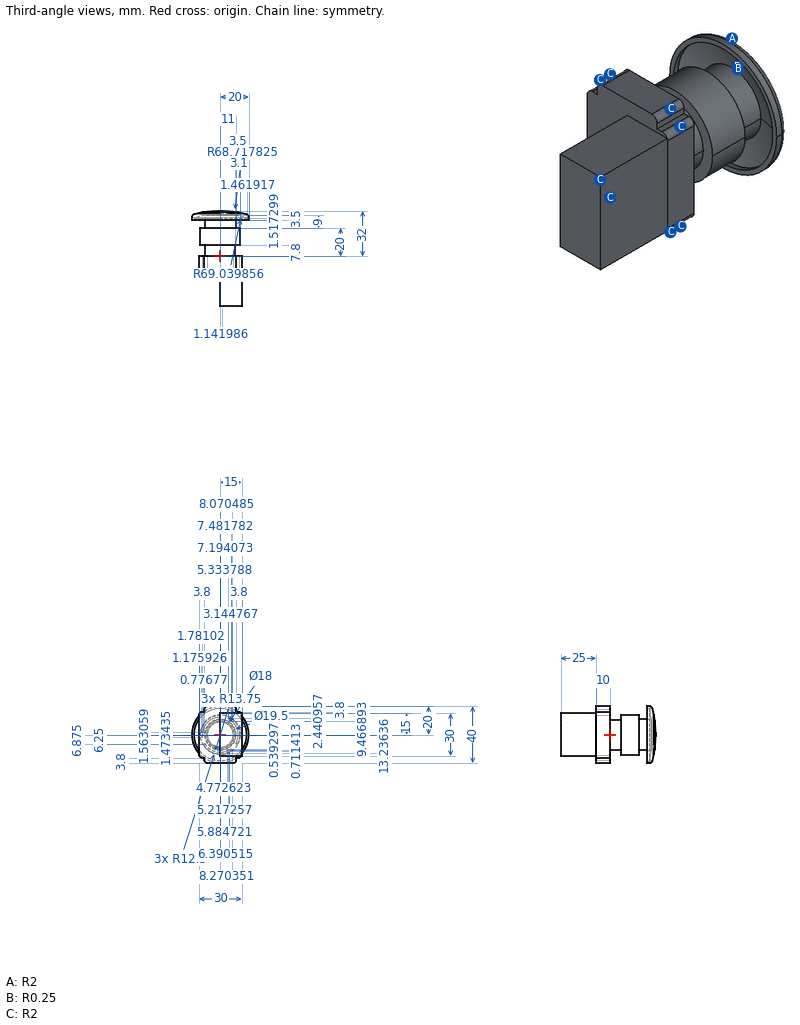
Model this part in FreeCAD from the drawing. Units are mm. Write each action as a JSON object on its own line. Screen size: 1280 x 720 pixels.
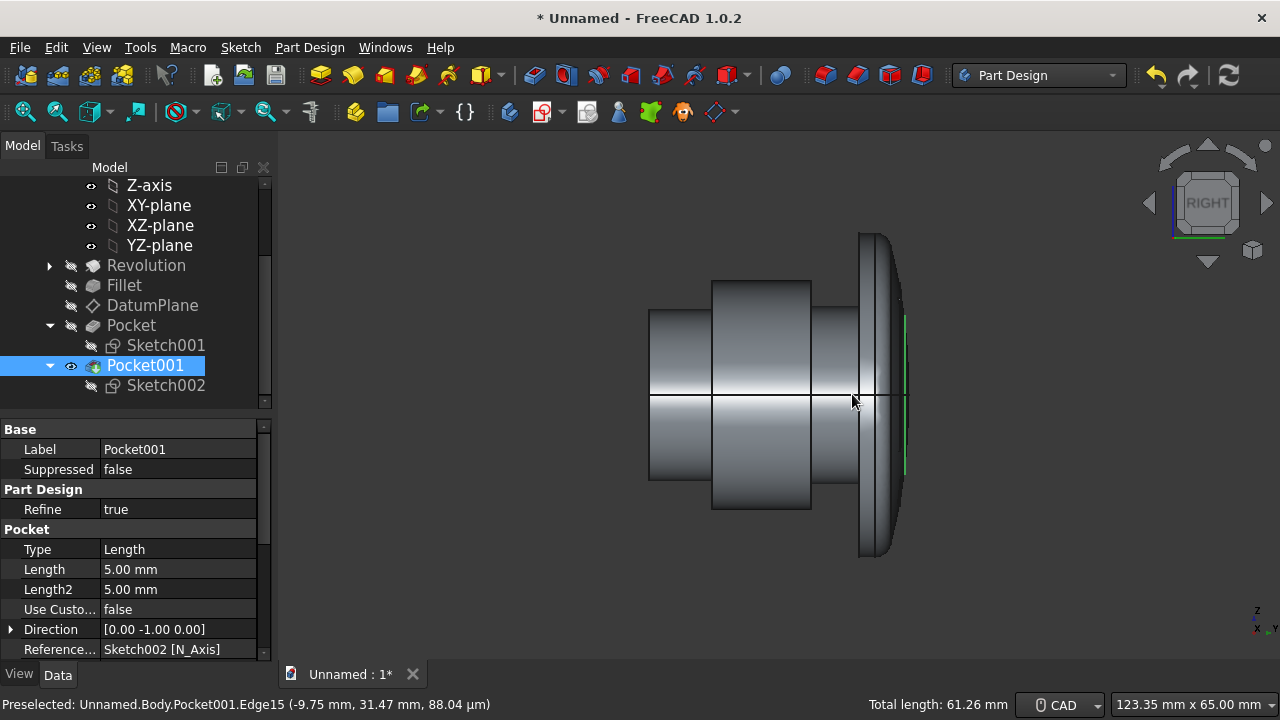
{"action": "key", "text": "5"}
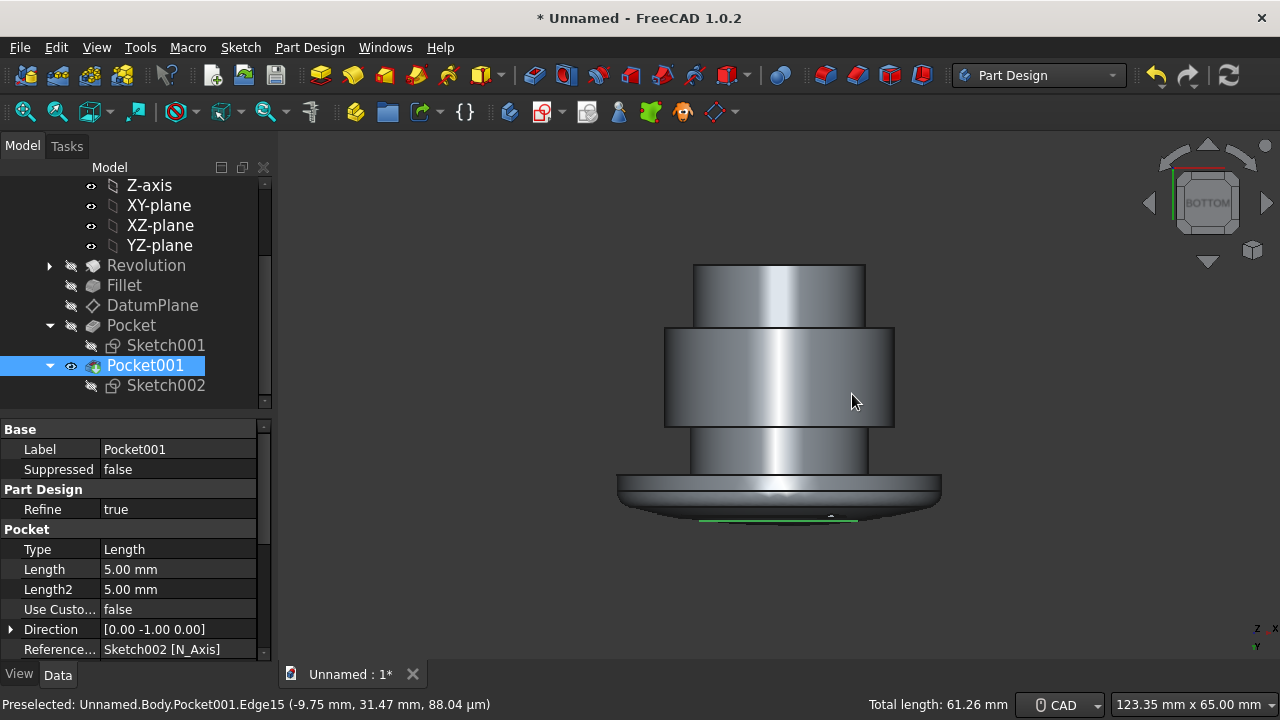
{"action": "key", "text": "4"}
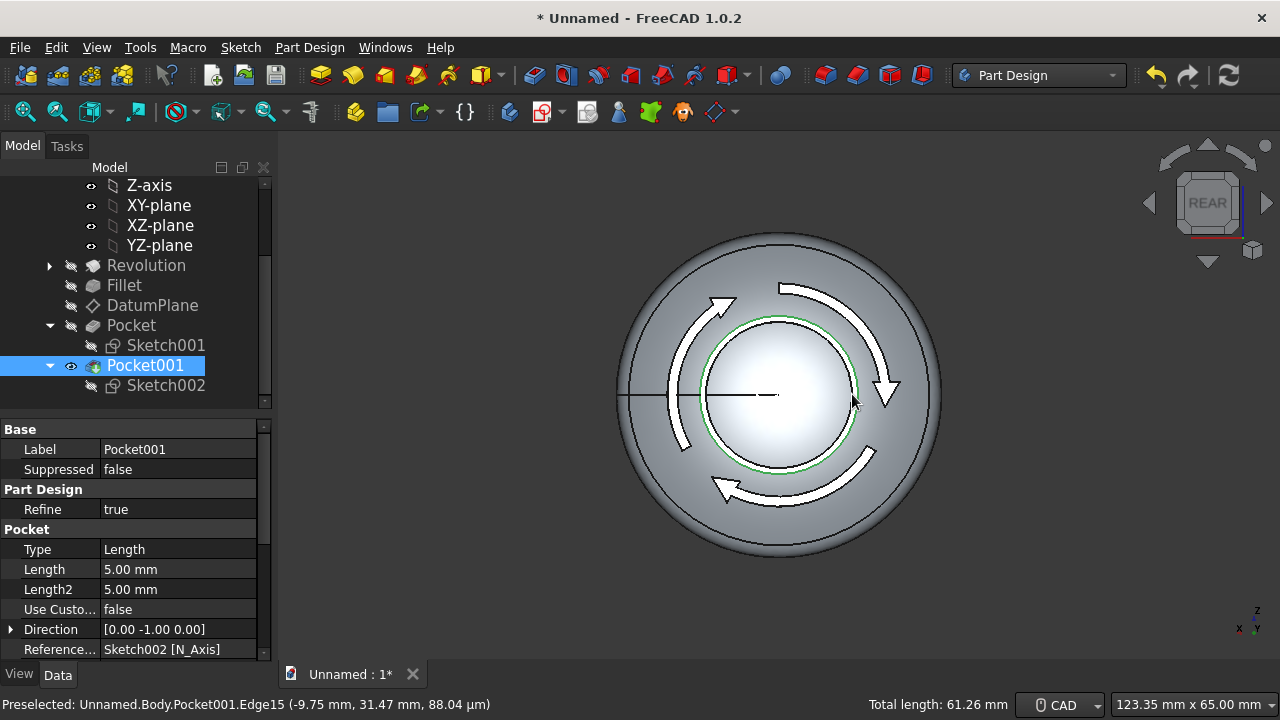
{"action": "key", "text": "6"}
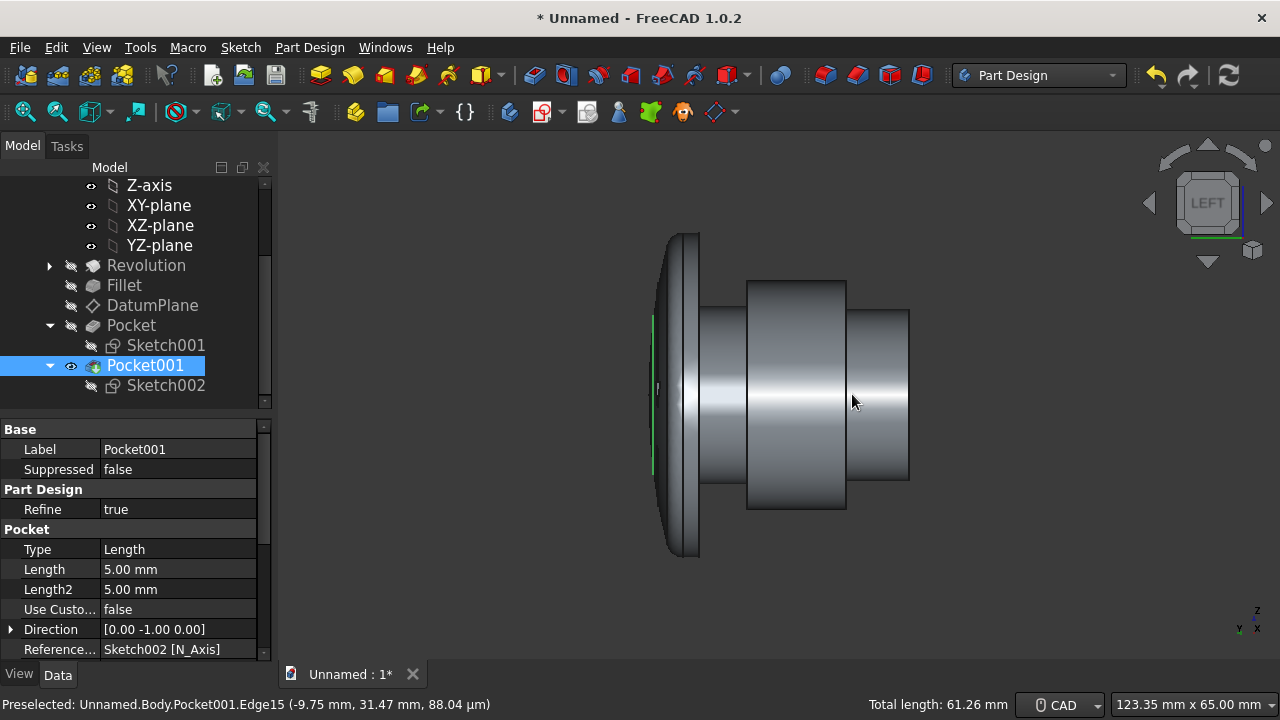
{"action": "key", "text": "v 3"}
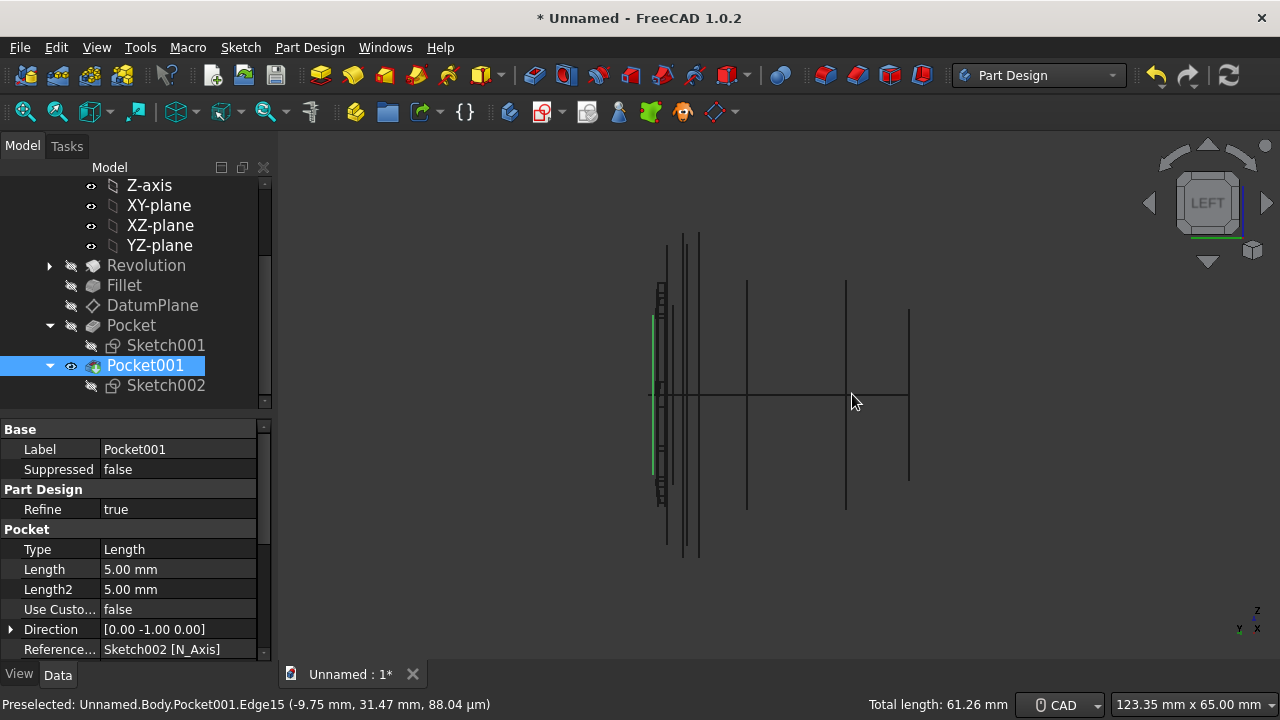
{"action": "key", "text": "0"}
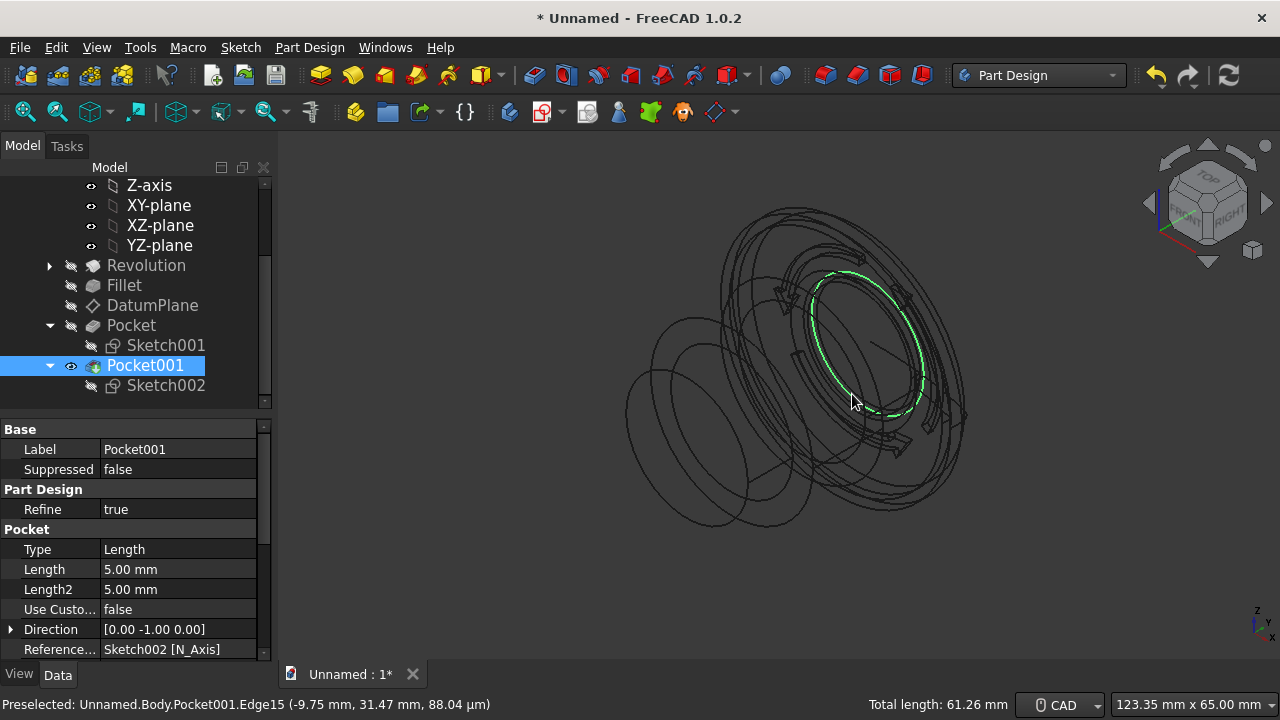
{"action": "left_click", "coordinate": [827, 353], "text": "ctrl"}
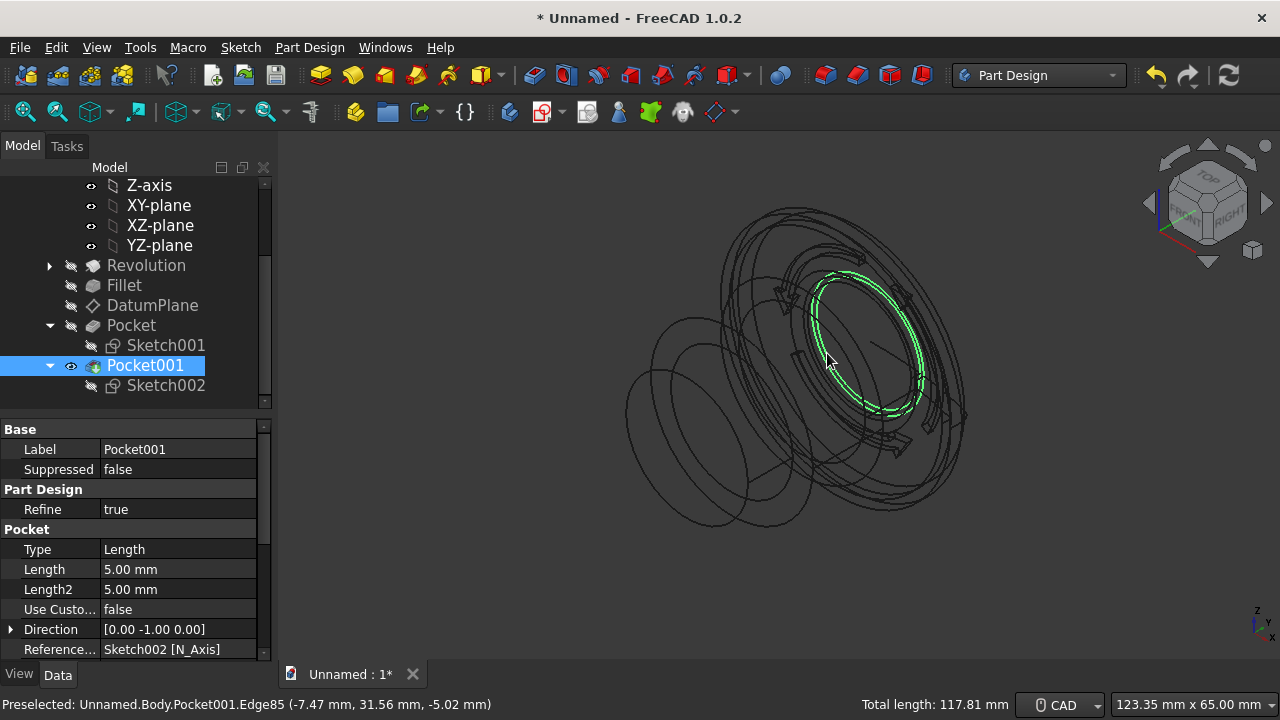
{"action": "key", "text": "v 1"}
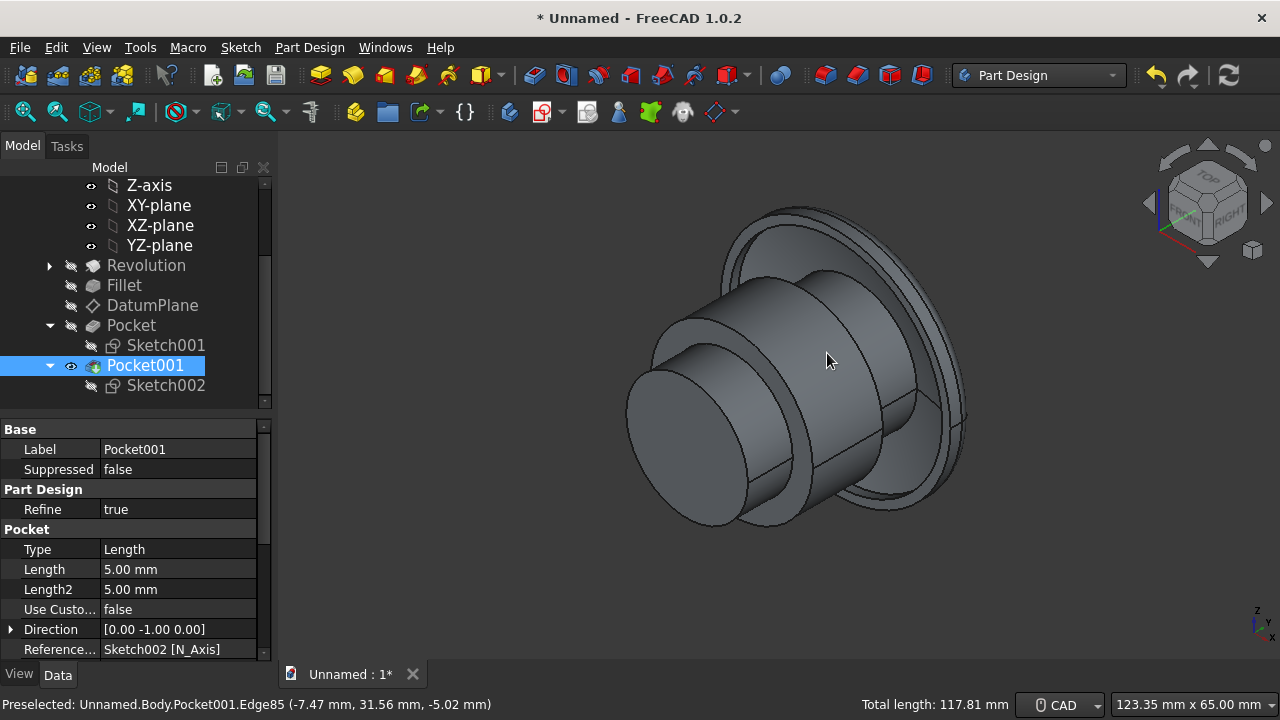
{"action": "left_click", "coordinate": [826, 76]}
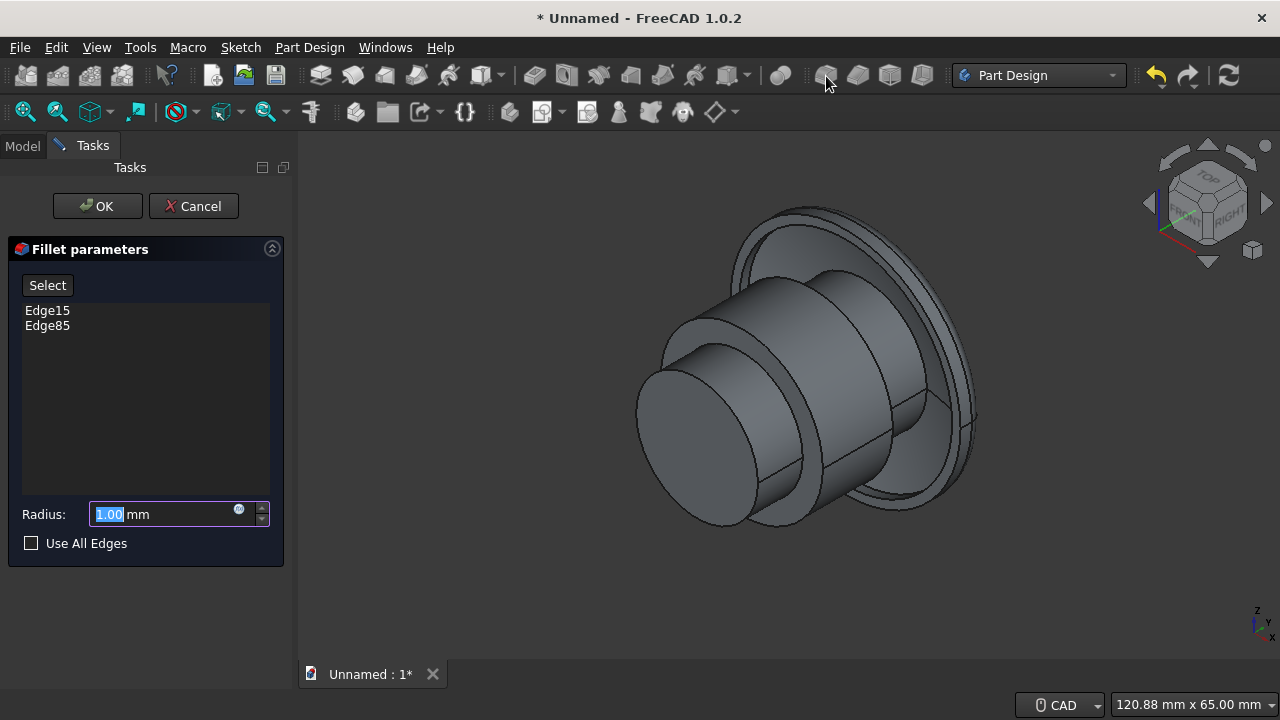
{"action": "type", "text": "0.25"}
{"action": "key", "text": "Tab"}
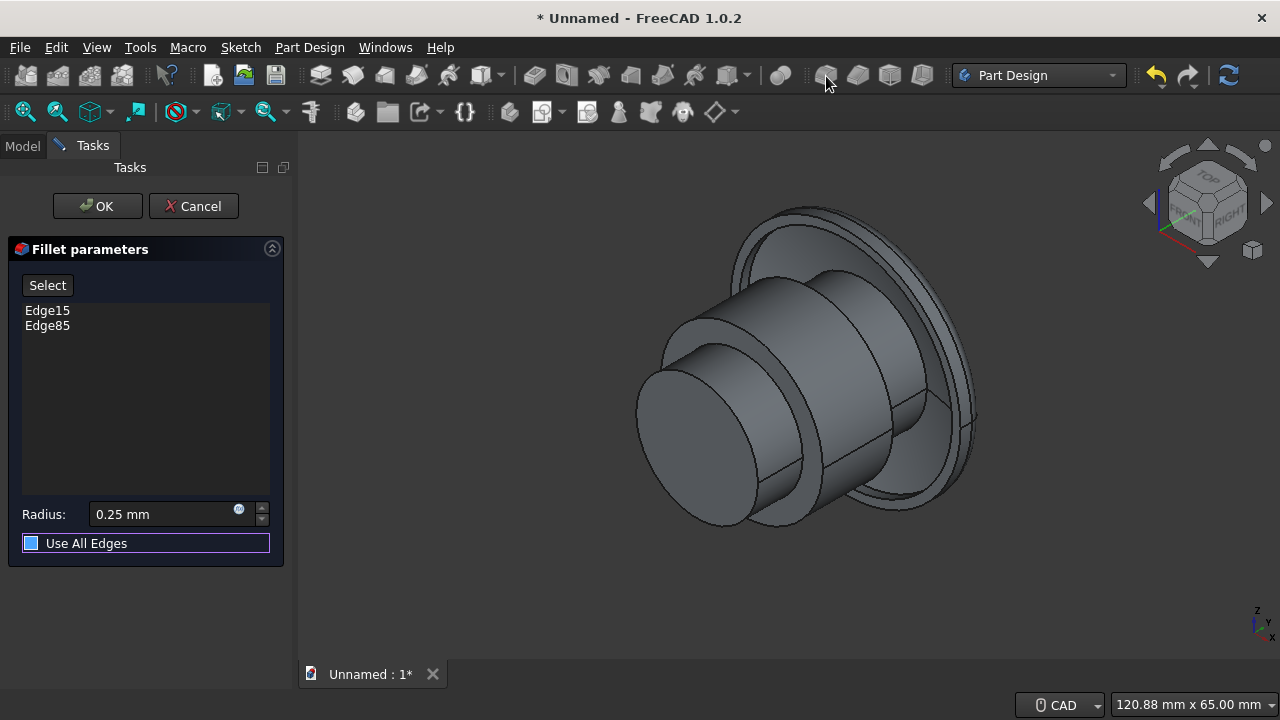
{"action": "left_click", "coordinate": [98, 206]}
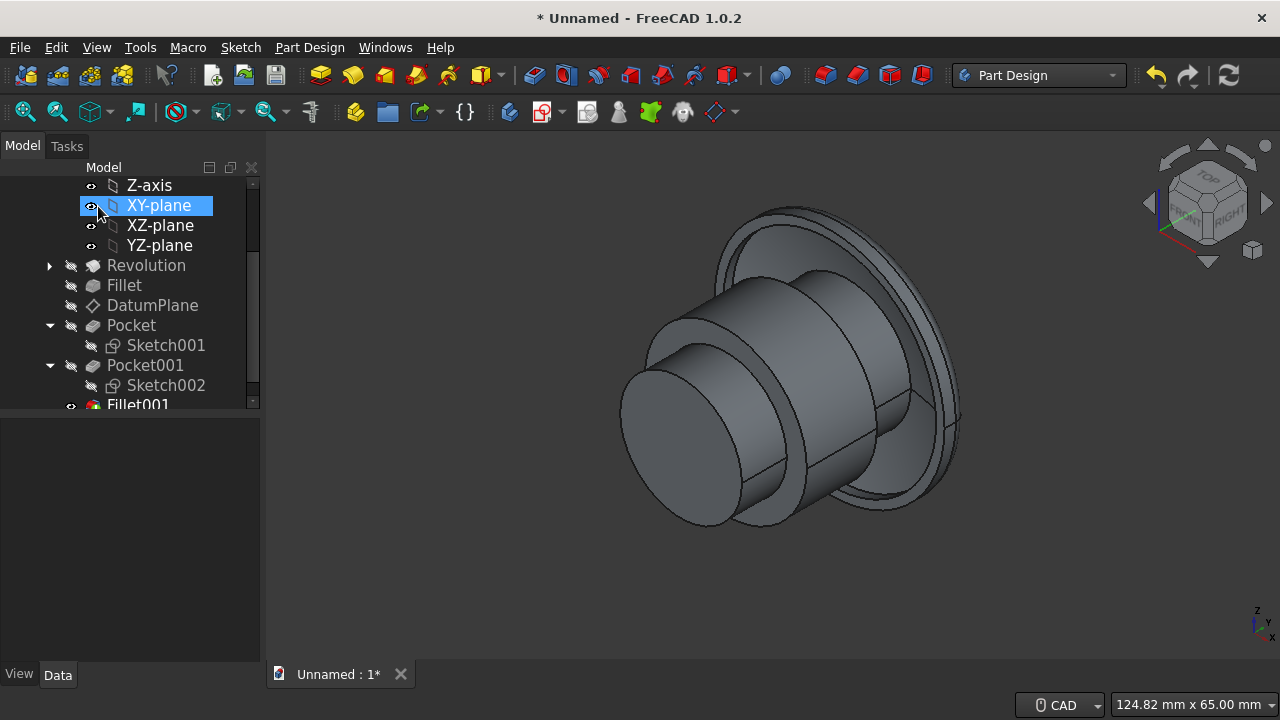
{"action": "left_click", "coordinate": [510, 112]}